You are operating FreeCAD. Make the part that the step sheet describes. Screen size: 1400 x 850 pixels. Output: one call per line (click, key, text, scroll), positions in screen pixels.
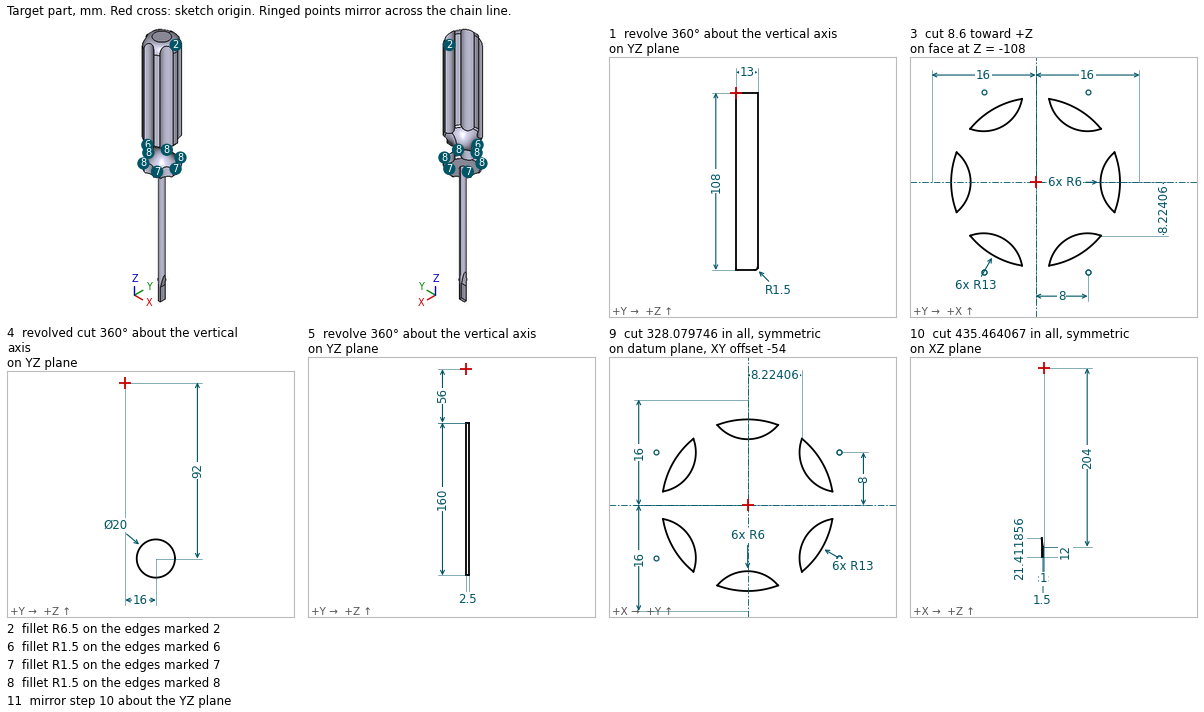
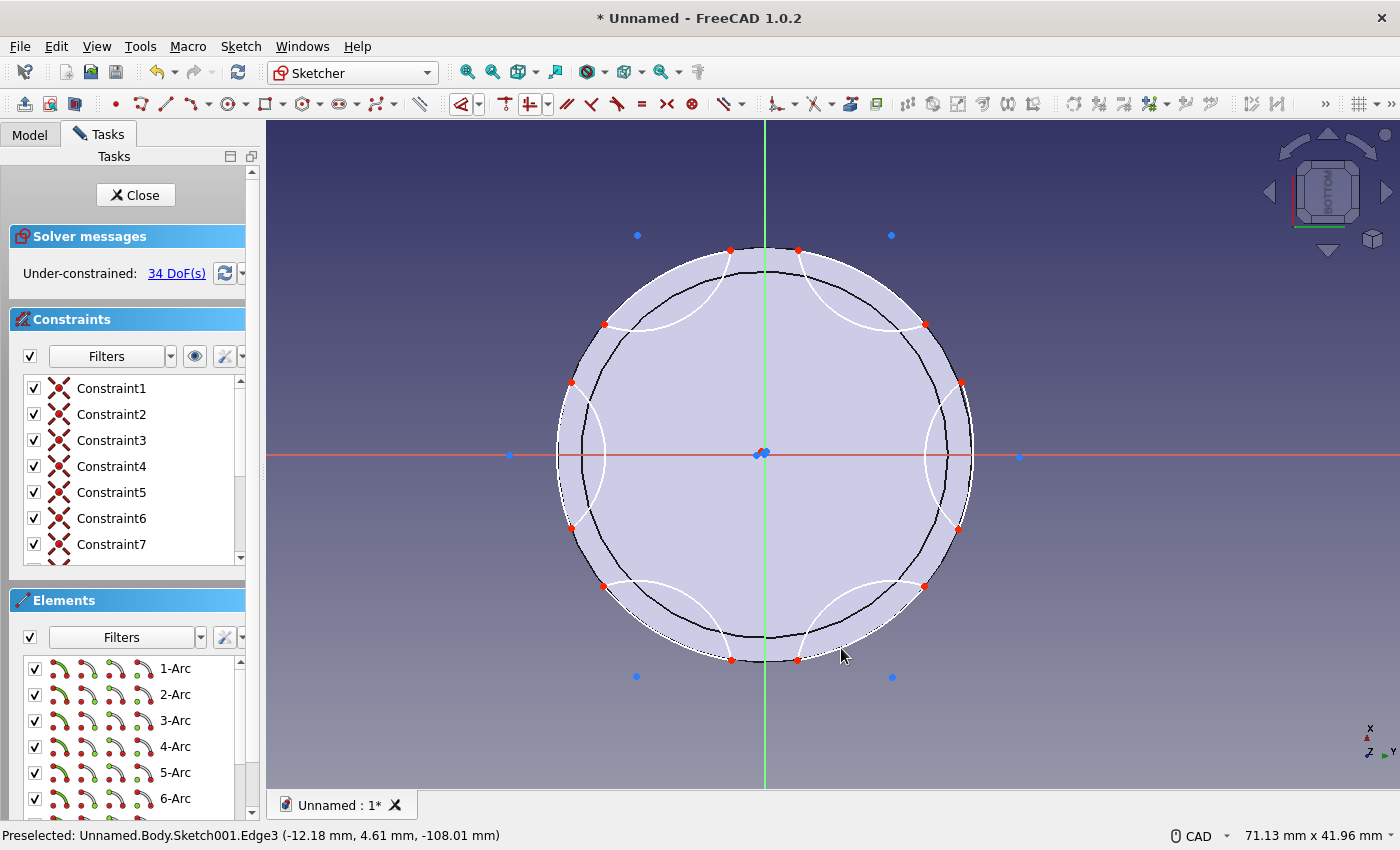
click(971, 486)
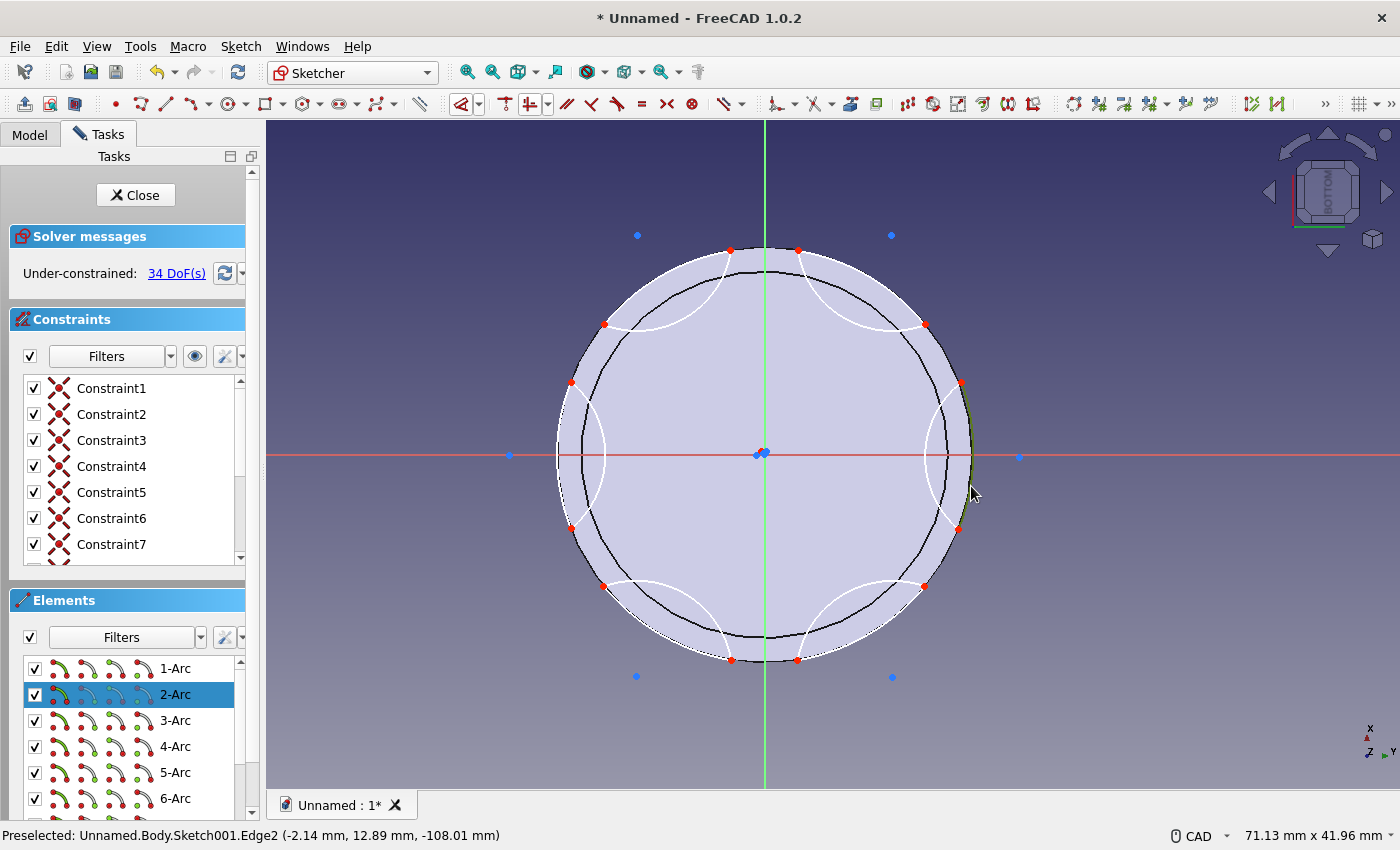
click(636, 618)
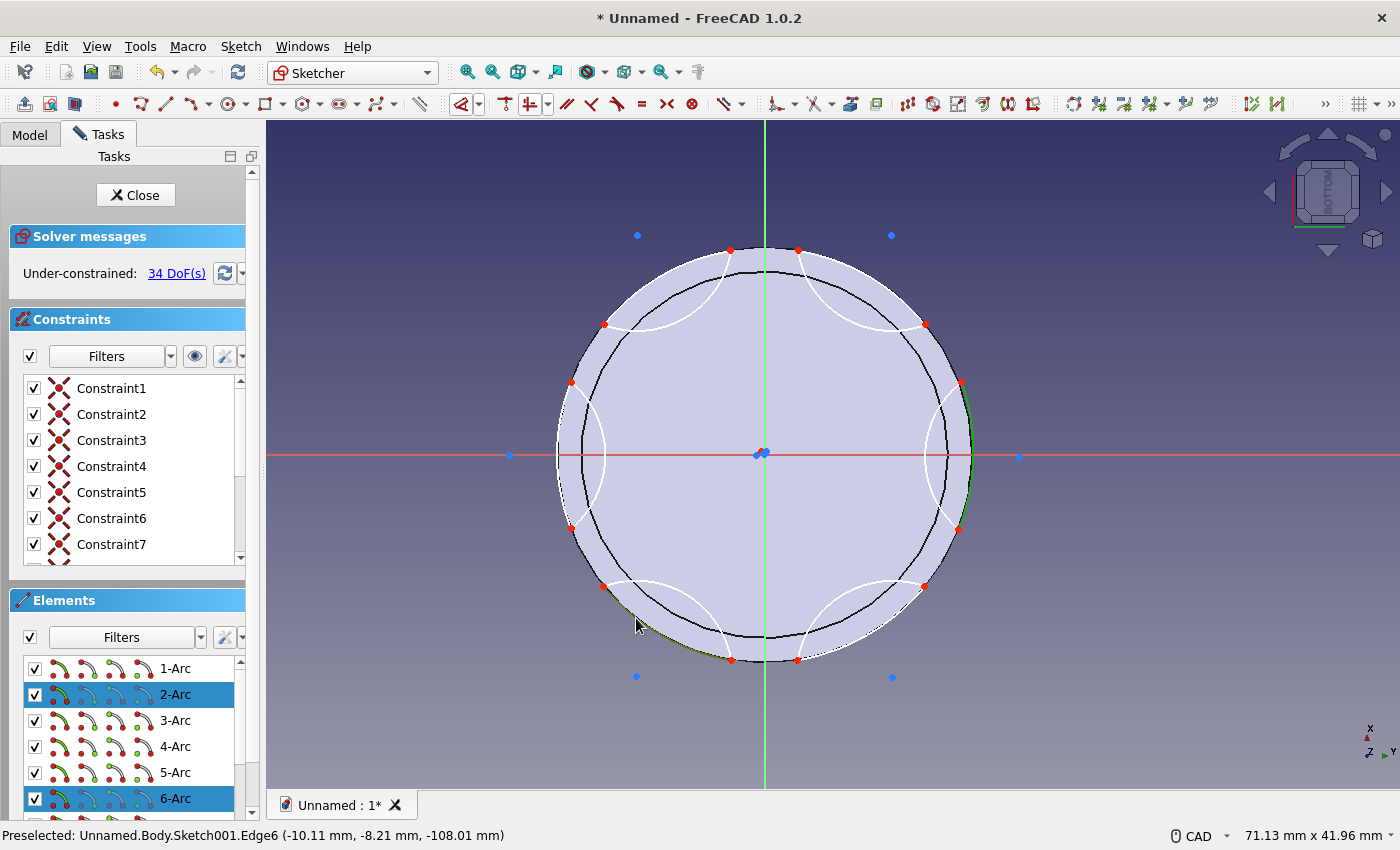
key(c)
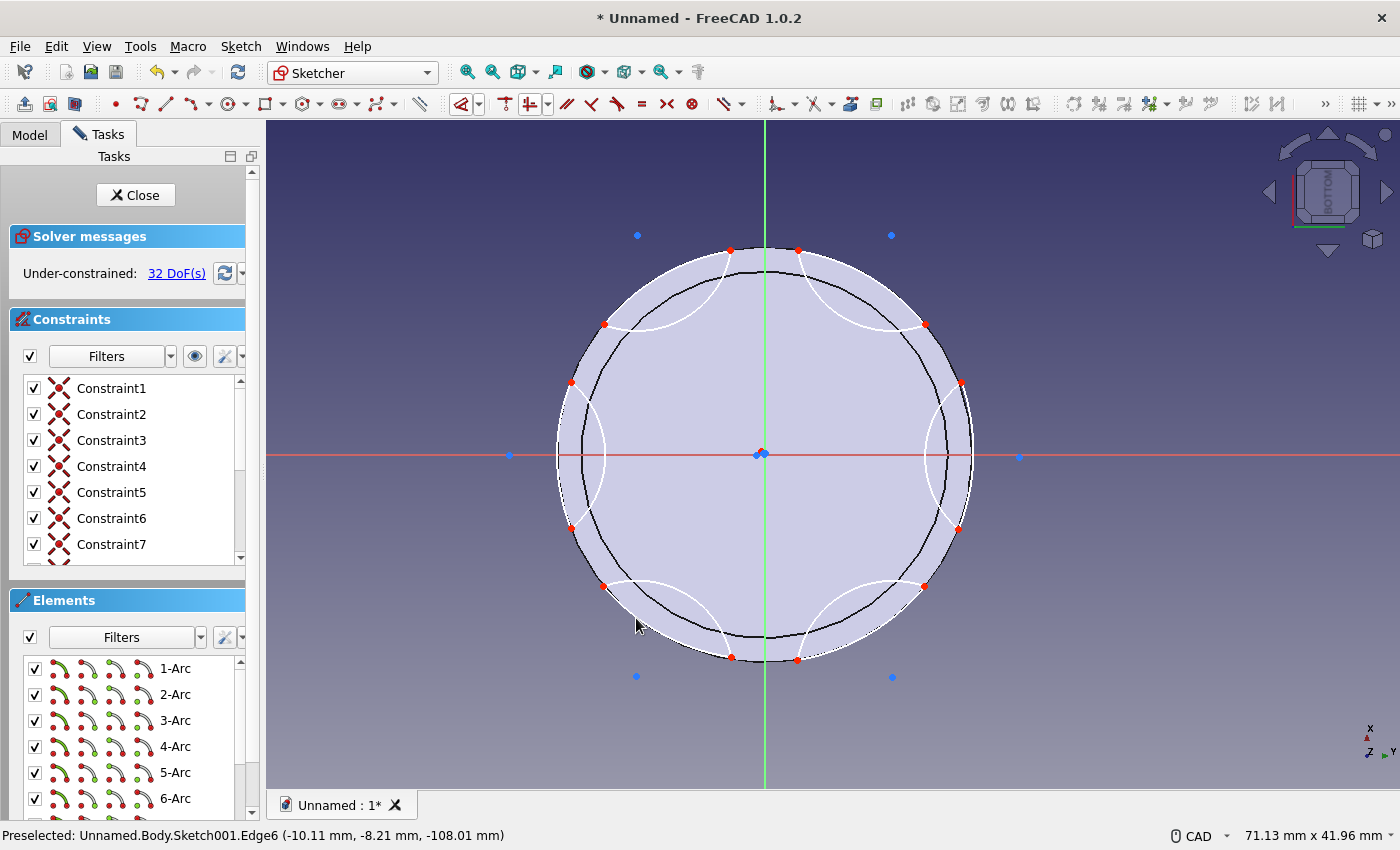
click(971, 486)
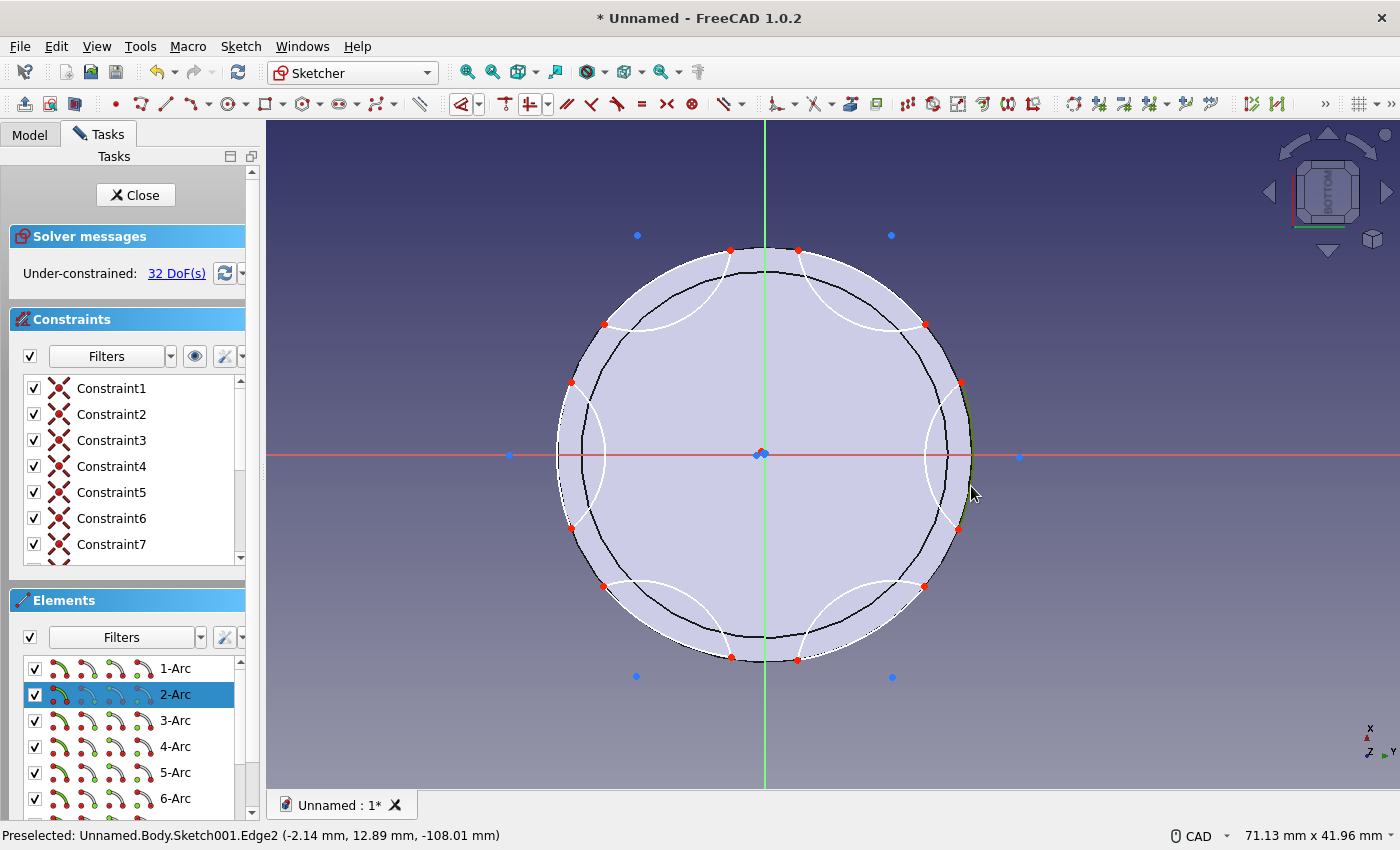
click(559, 425)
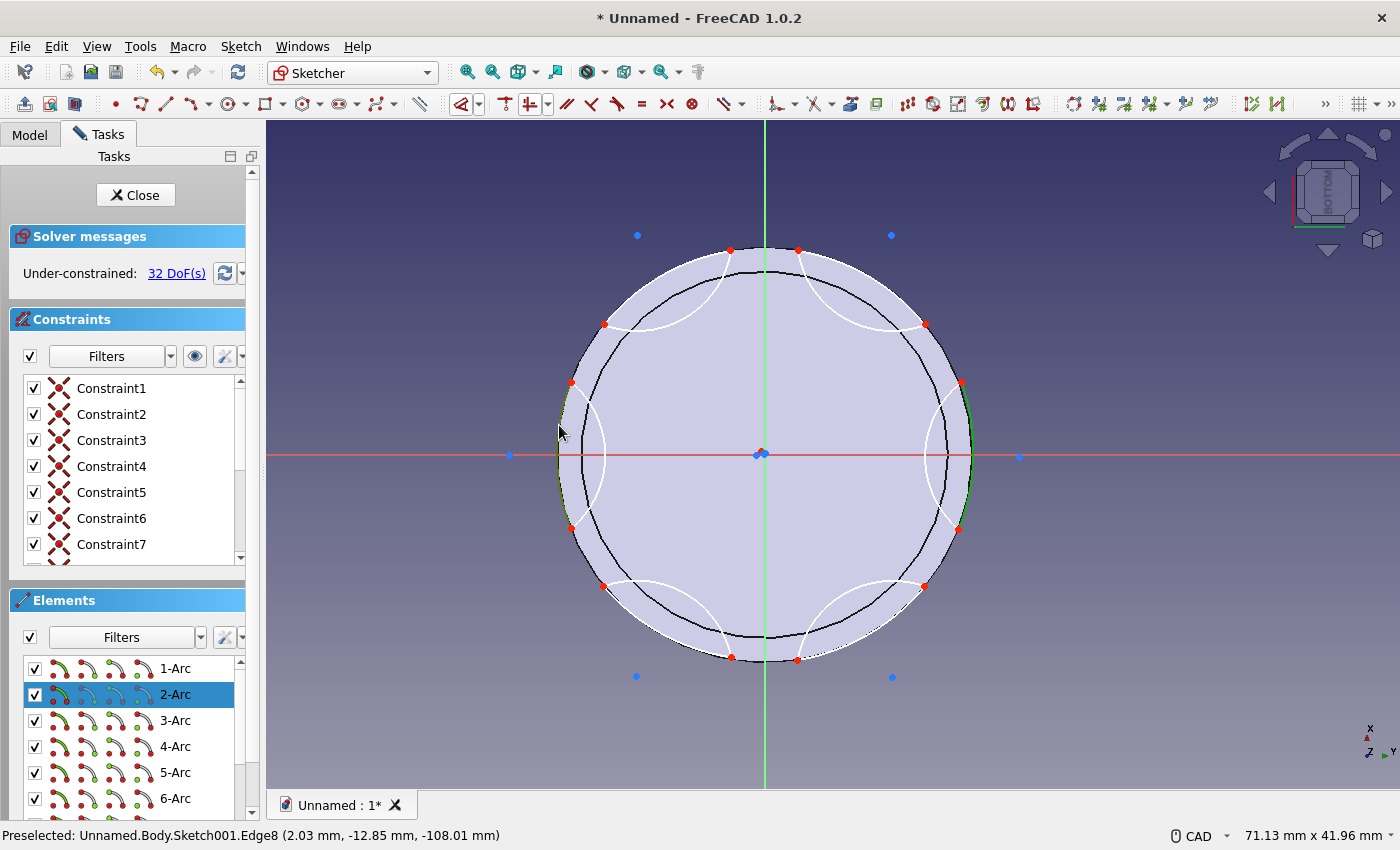
click(505, 104)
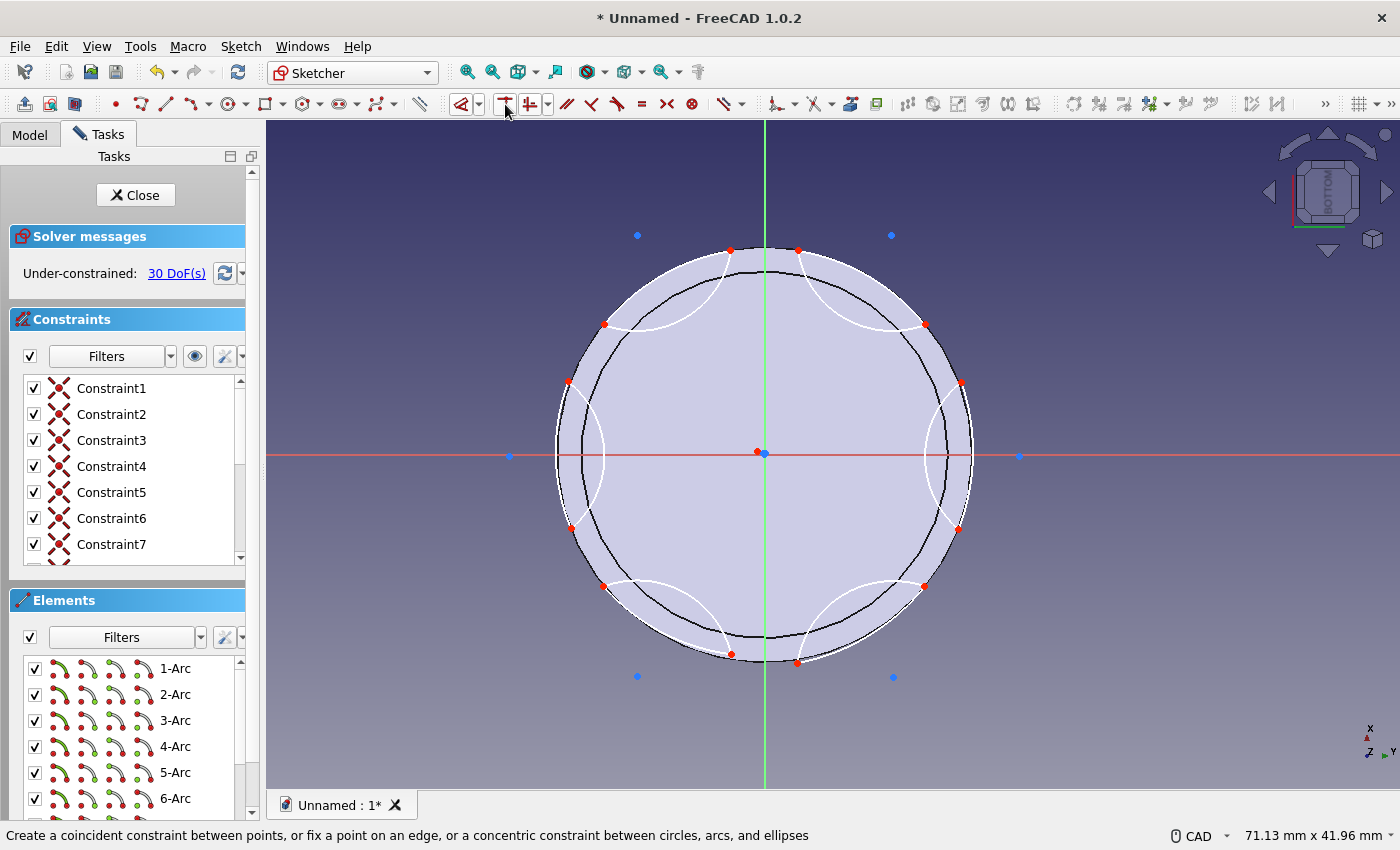
click(970, 486)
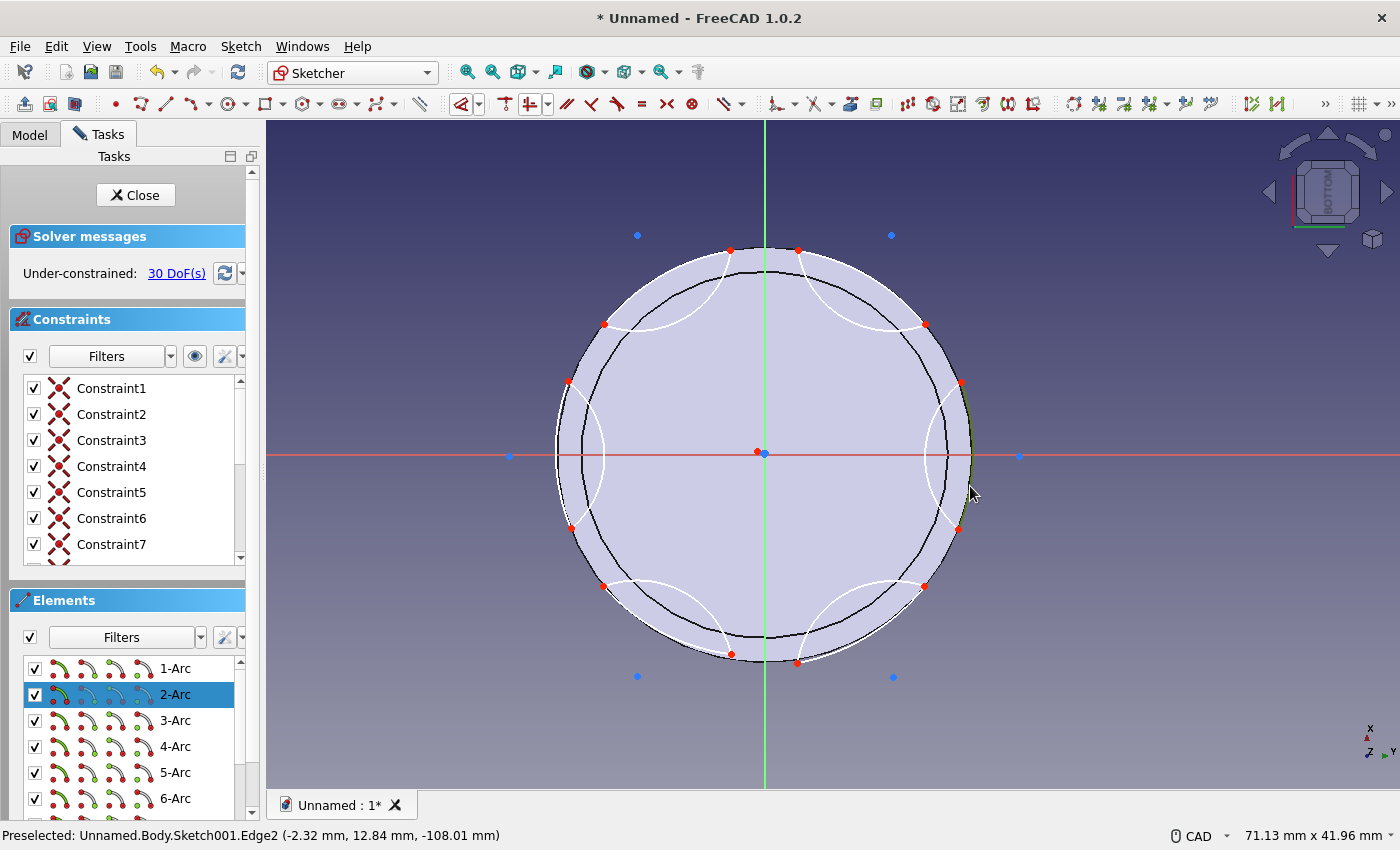
click(688, 263)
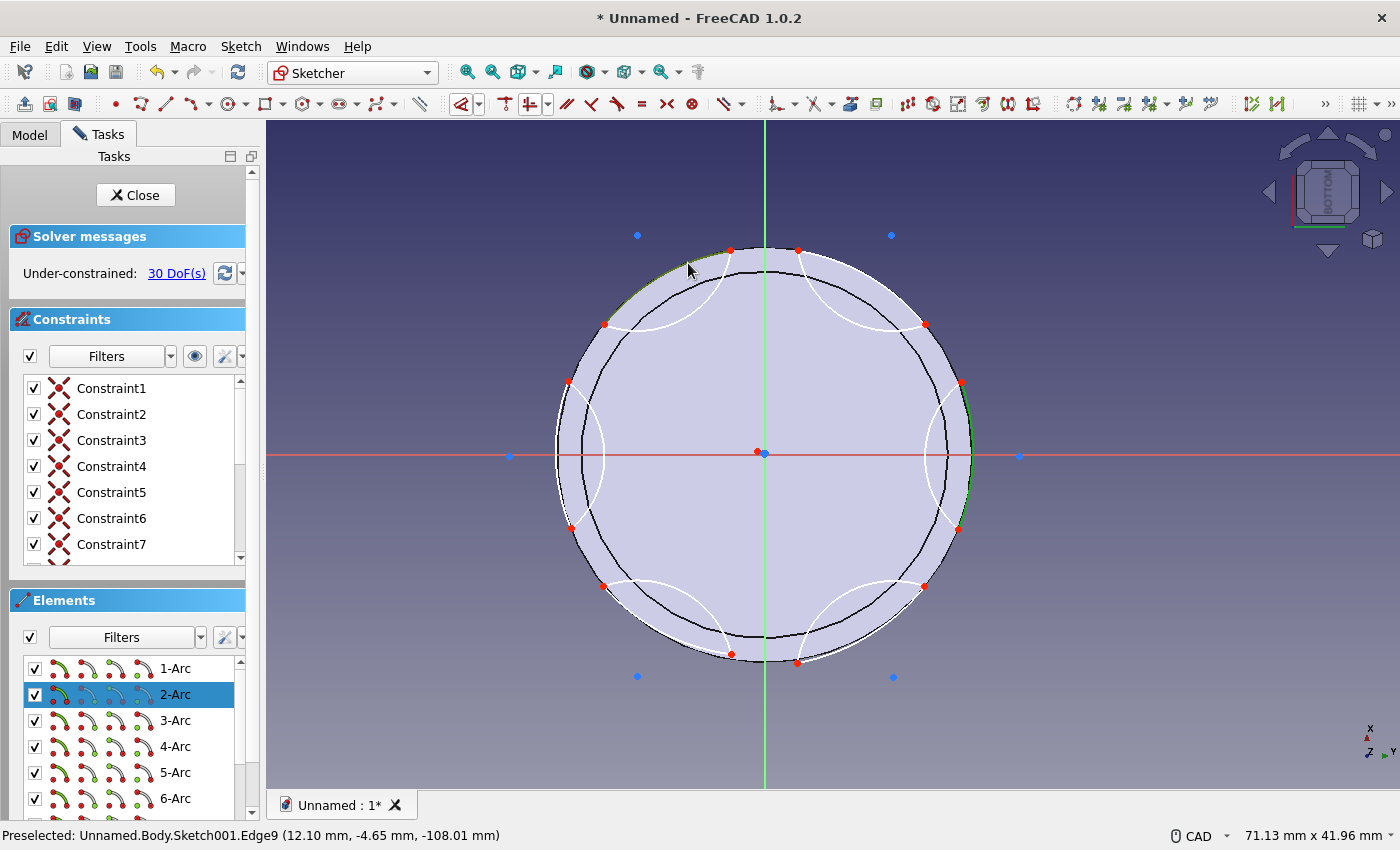
click(505, 104)